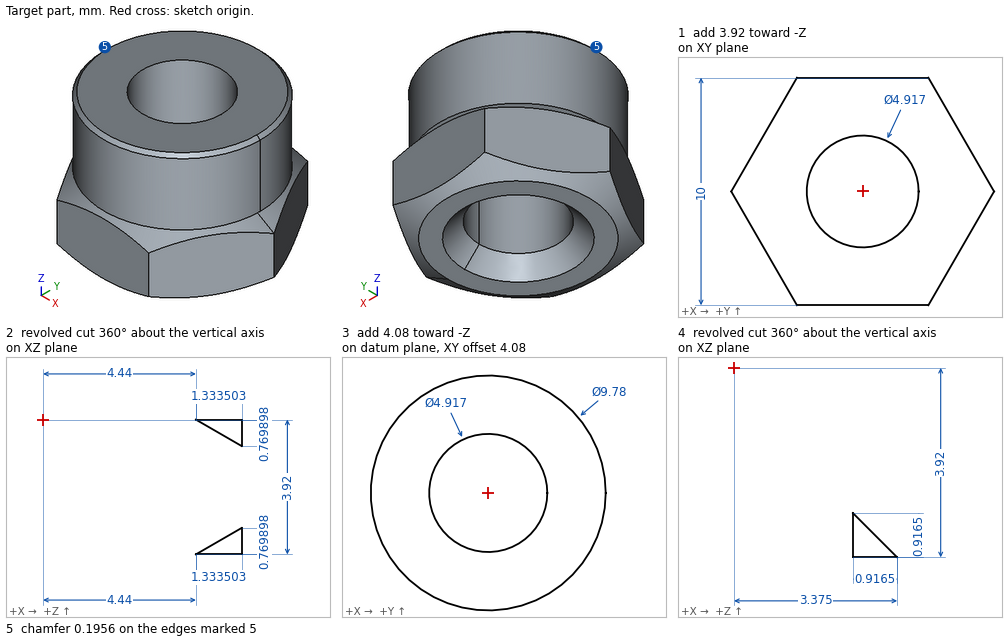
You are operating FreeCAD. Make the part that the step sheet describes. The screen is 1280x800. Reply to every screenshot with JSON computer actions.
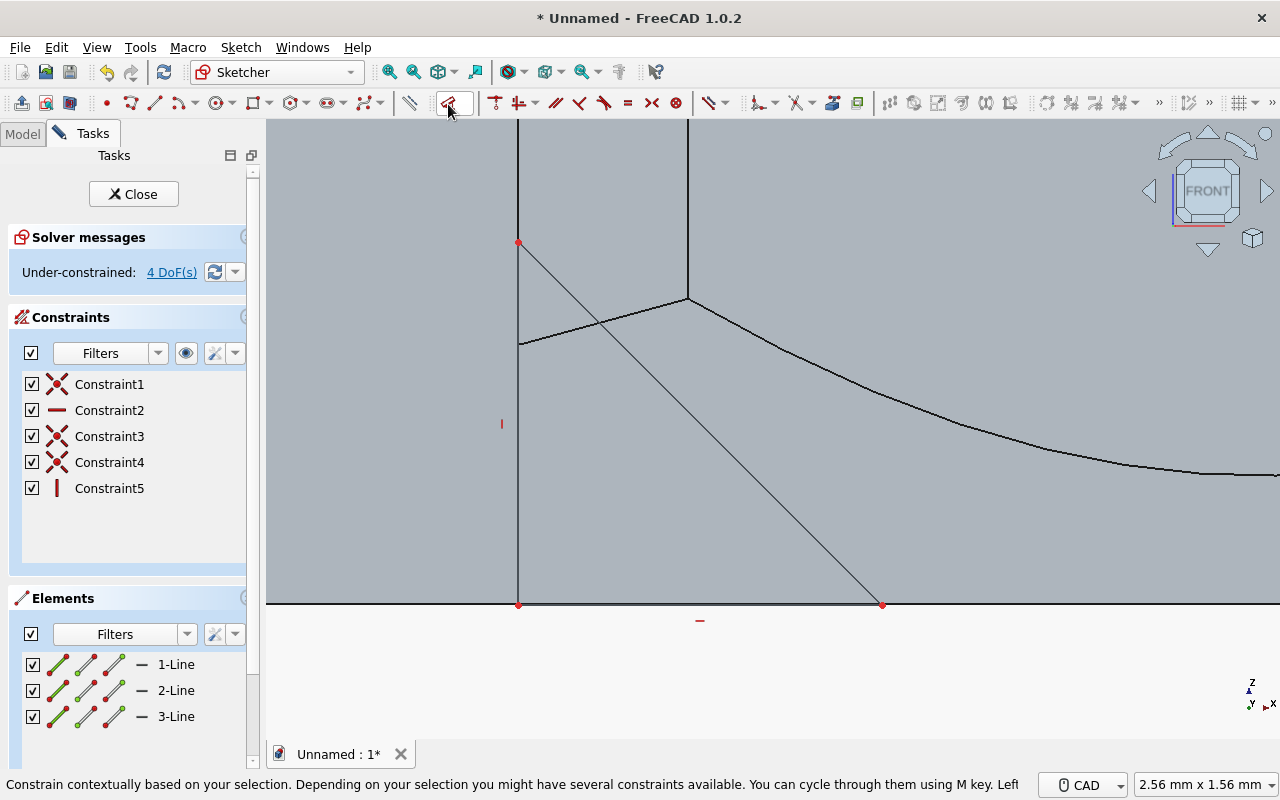
{"action": "left_click", "coordinate": [882, 605]}
{"action": "left_click", "coordinate": [916, 376]}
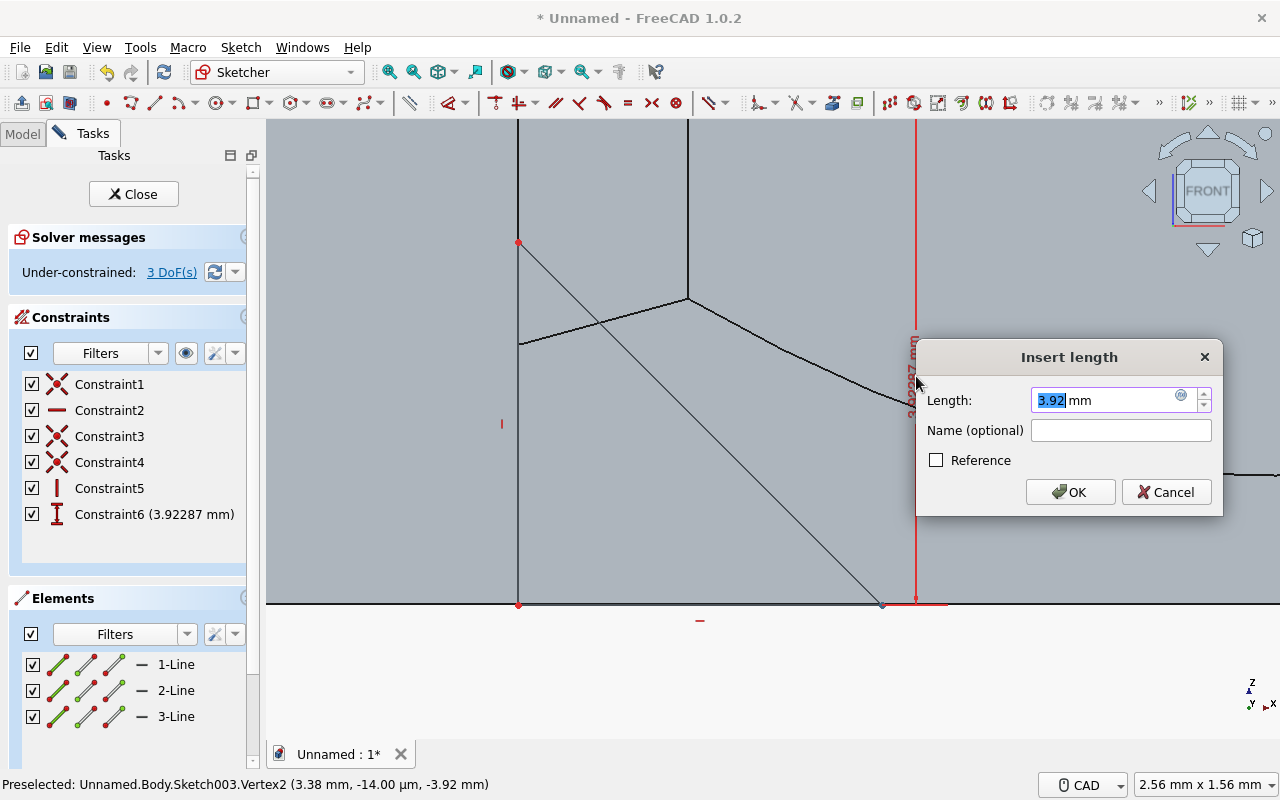
{"action": "type", "text": "3.92"}
{"action": "key", "text": "Return"}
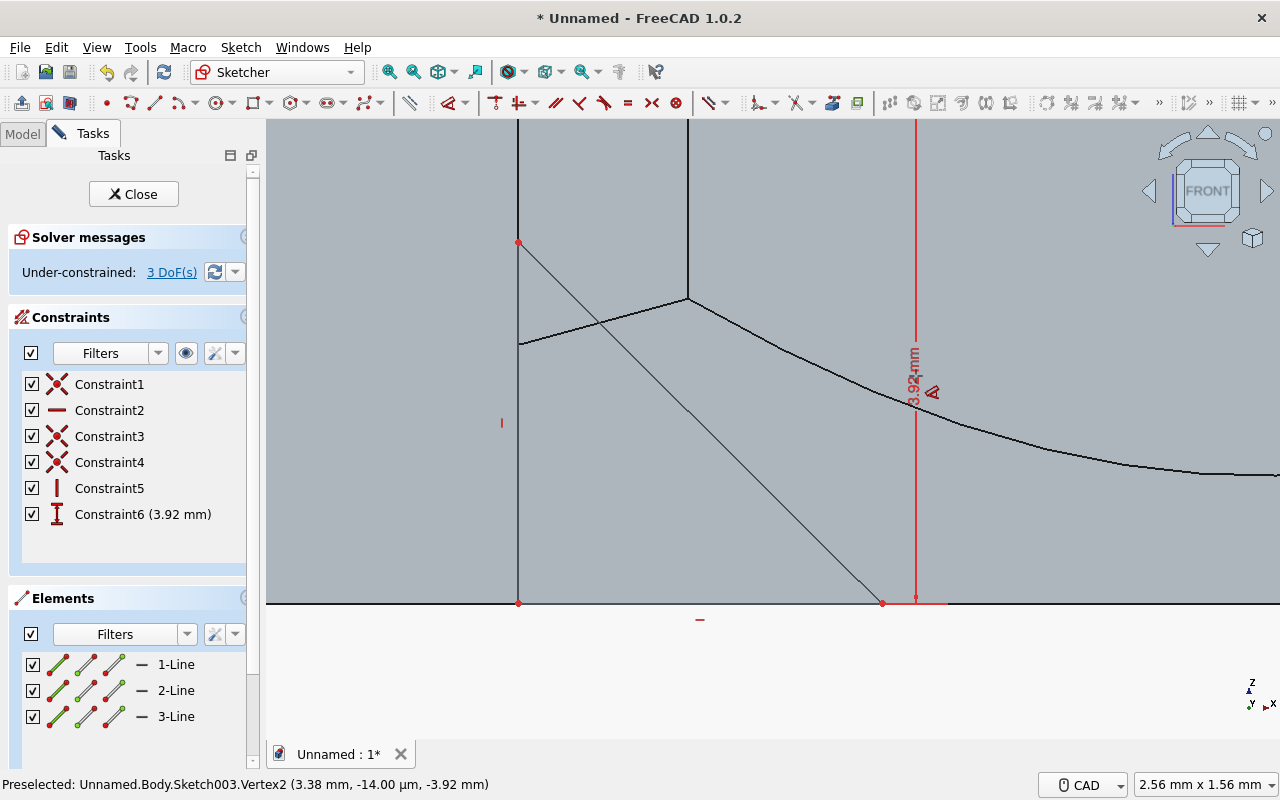
{"action": "left_click", "coordinate": [773, 604]}
{"action": "left_click", "coordinate": [700, 638]}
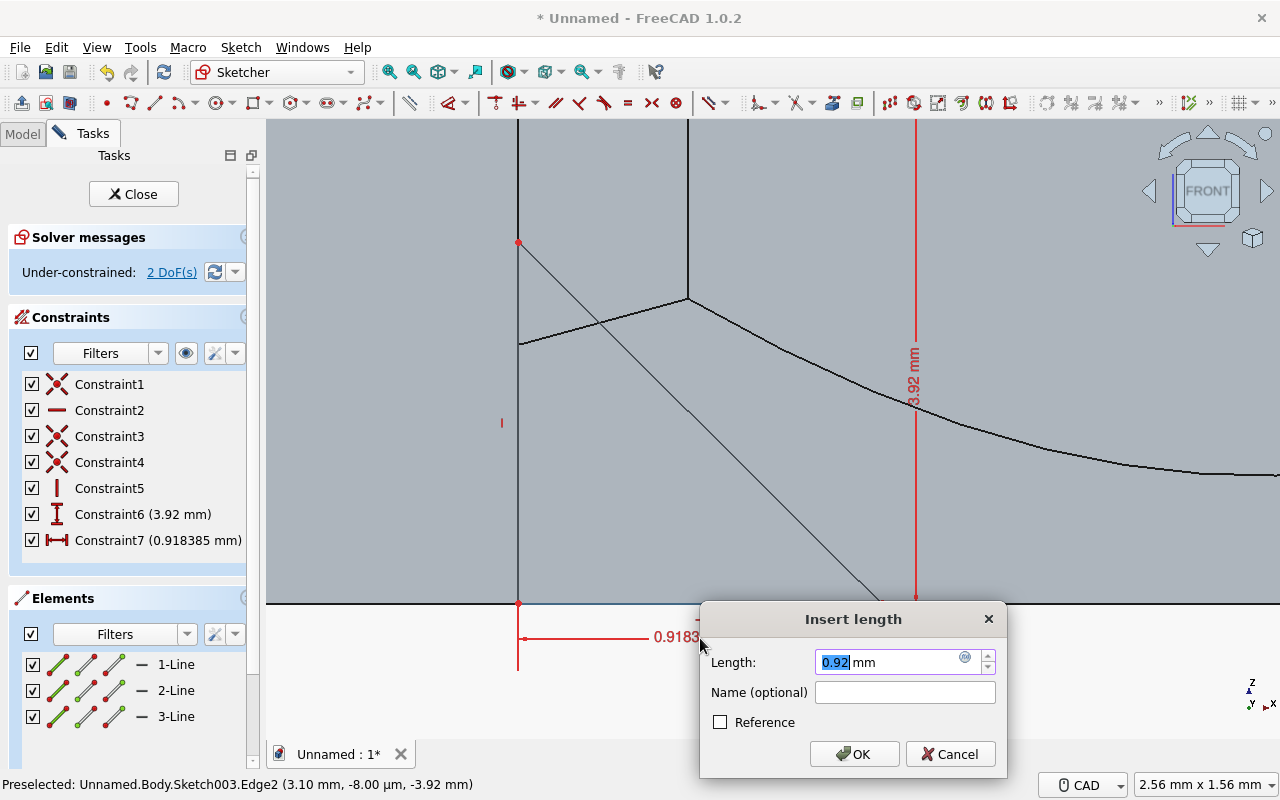
{"action": "type", "text": "0.9165"}
{"action": "key", "text": "Return"}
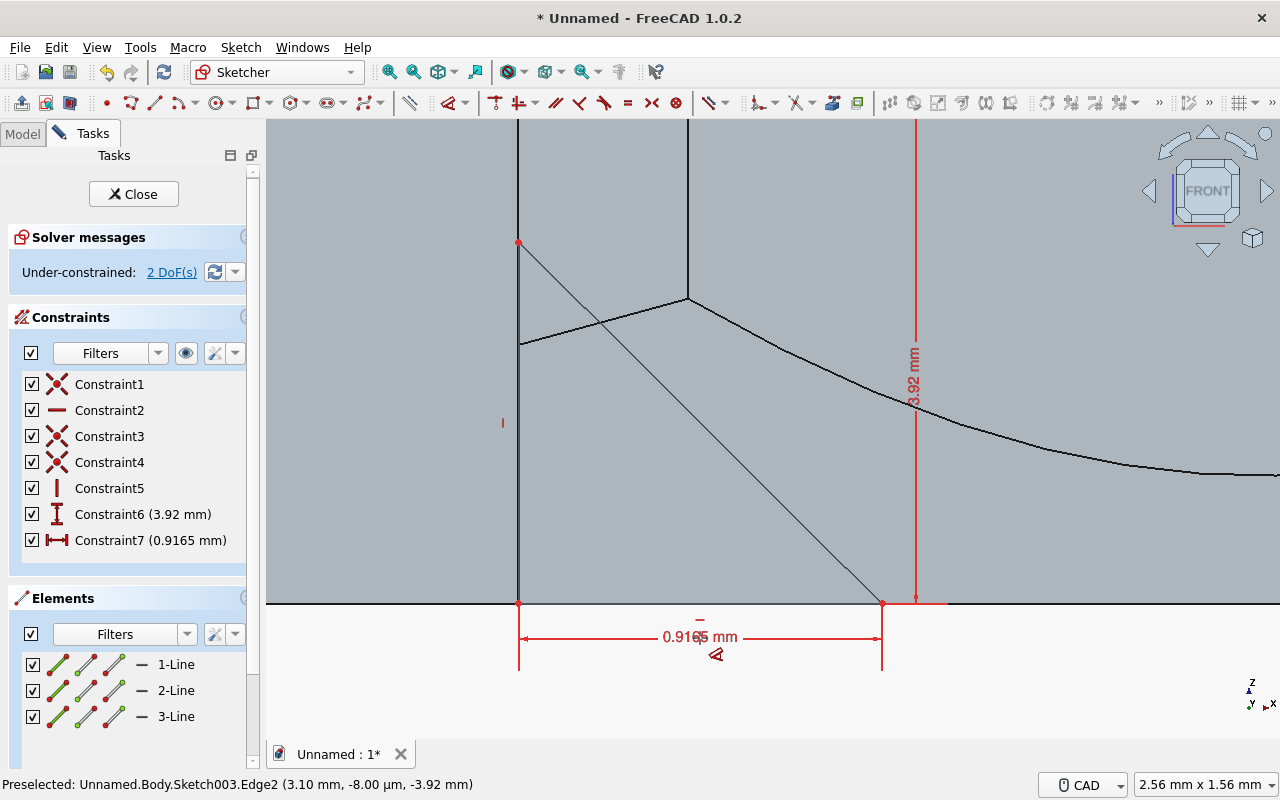
{"action": "left_click", "coordinate": [519, 495]}
{"action": "left_click", "coordinate": [485, 423]}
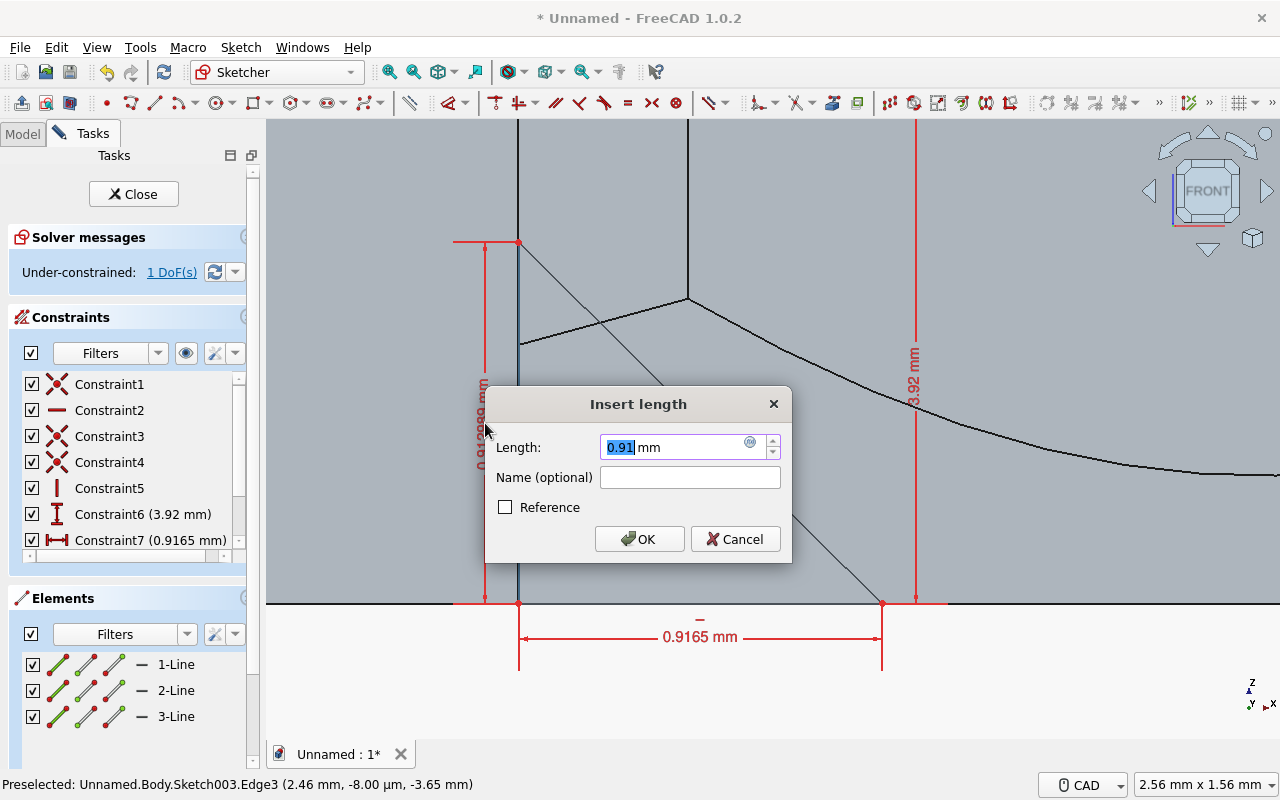
{"action": "type", "text": "0.9165"}
{"action": "key", "text": "Return"}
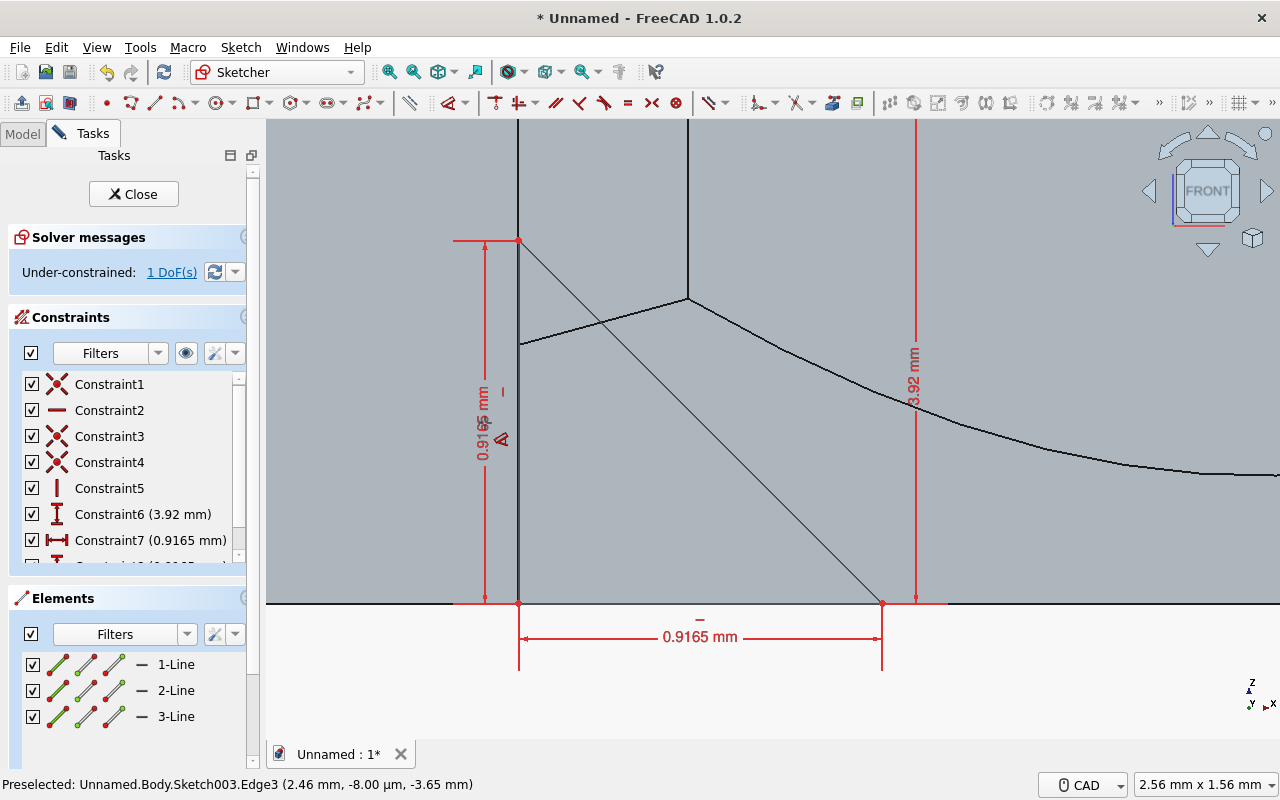
{"action": "left_click", "coordinate": [882, 604]}
{"action": "left_click", "coordinate": [588, 638]}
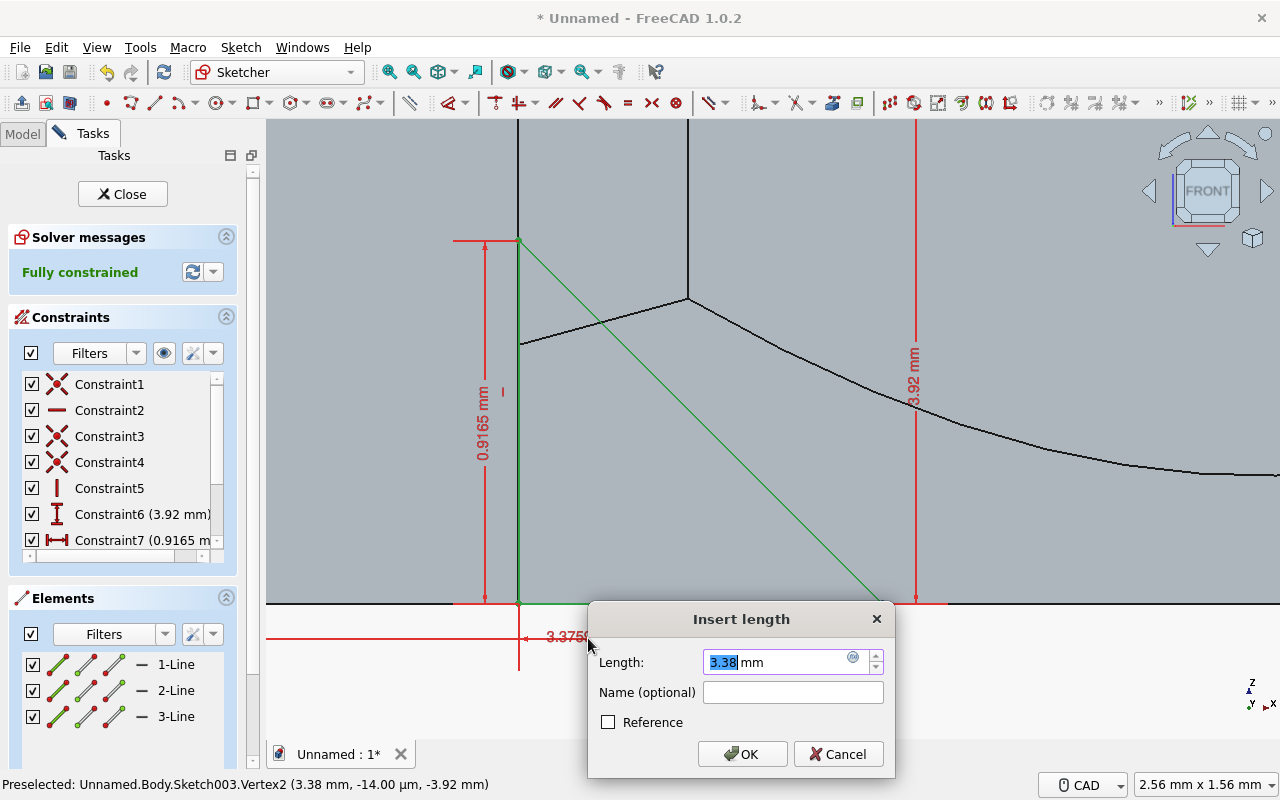
{"action": "type", "text": "3.375"}
{"action": "key", "text": "Return"}
{"action": "key", "text": "Escape"}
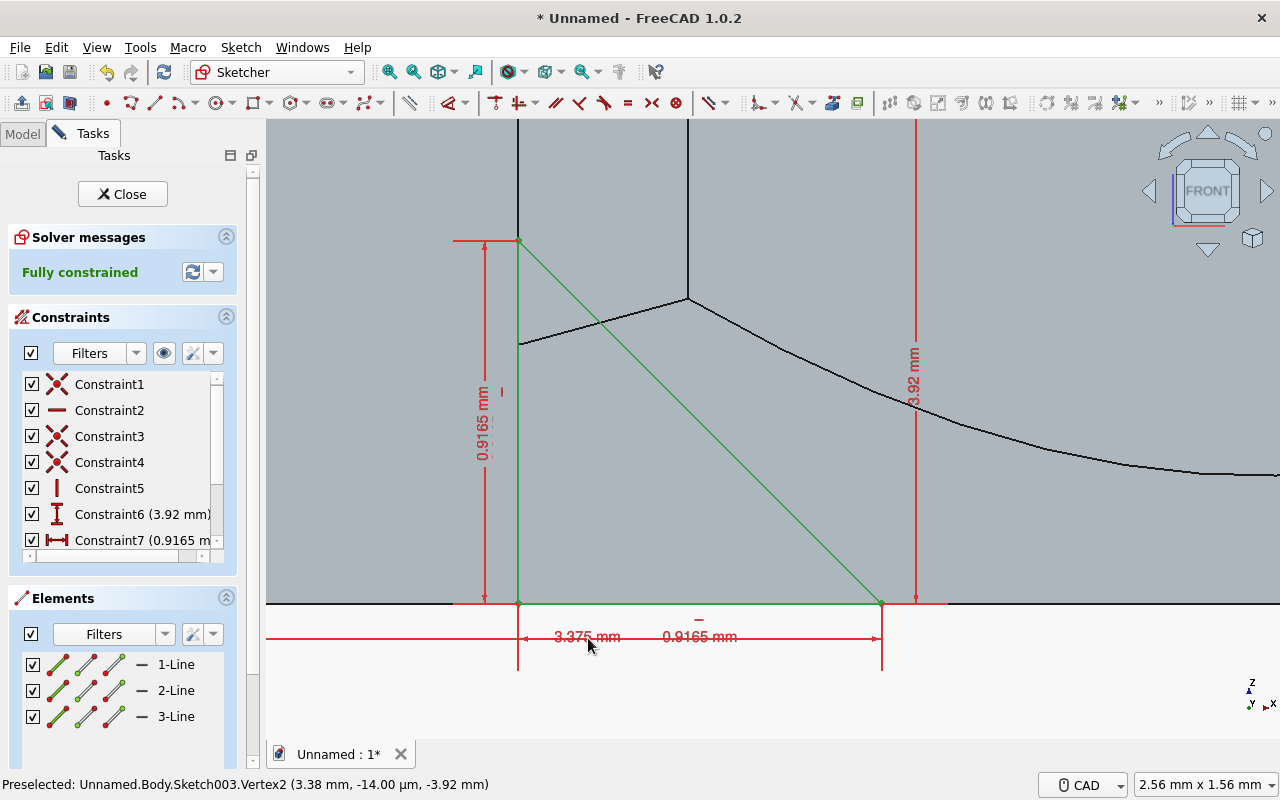
{"action": "left_click", "coordinate": [123, 194]}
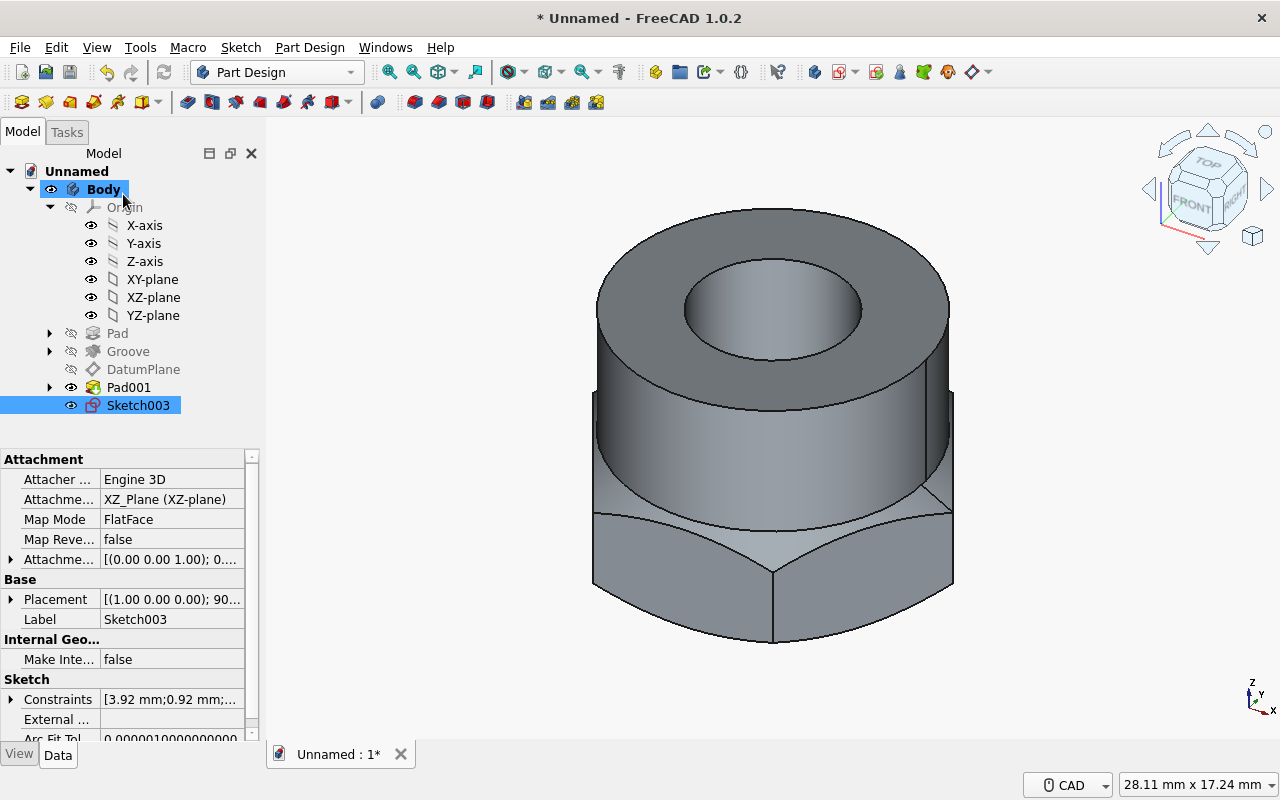
{"action": "left_click", "coordinate": [236, 102]}